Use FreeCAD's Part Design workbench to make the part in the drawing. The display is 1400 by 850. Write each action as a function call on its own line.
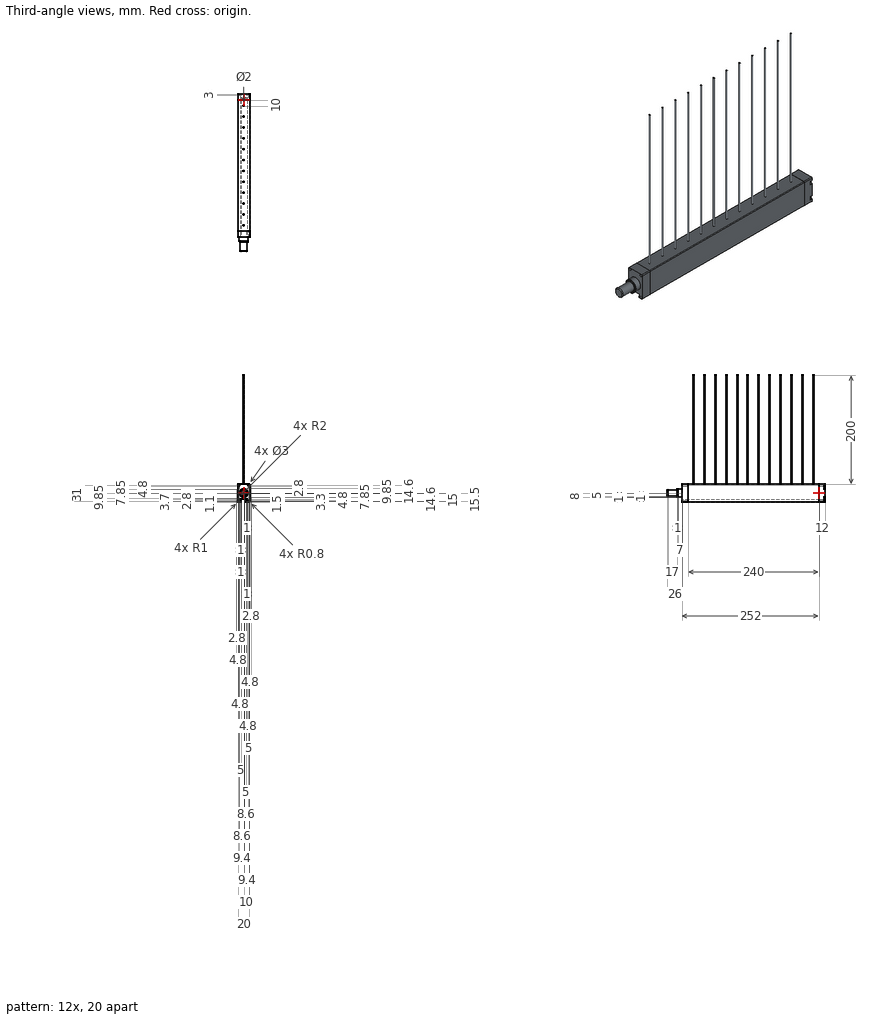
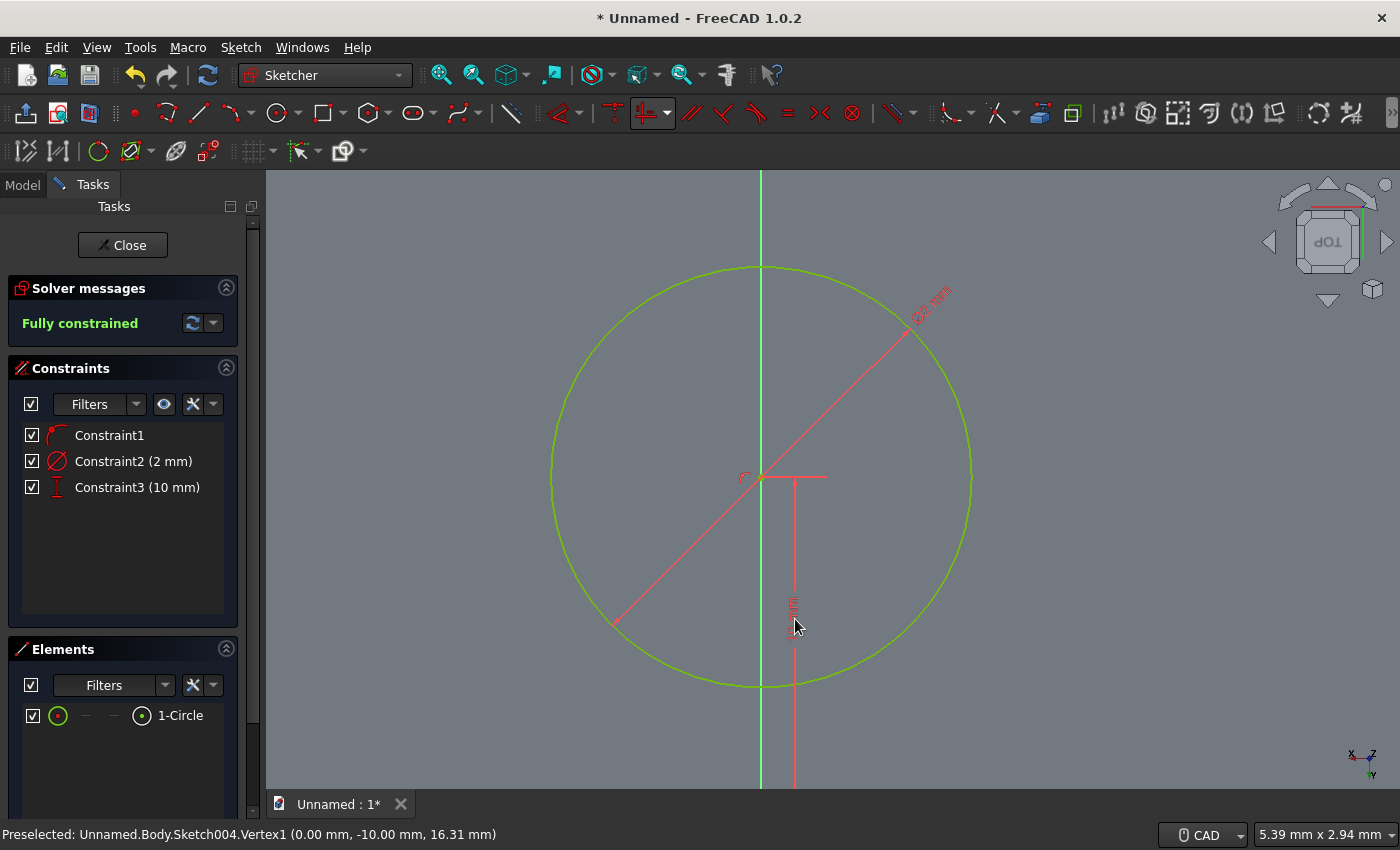
click(123, 245)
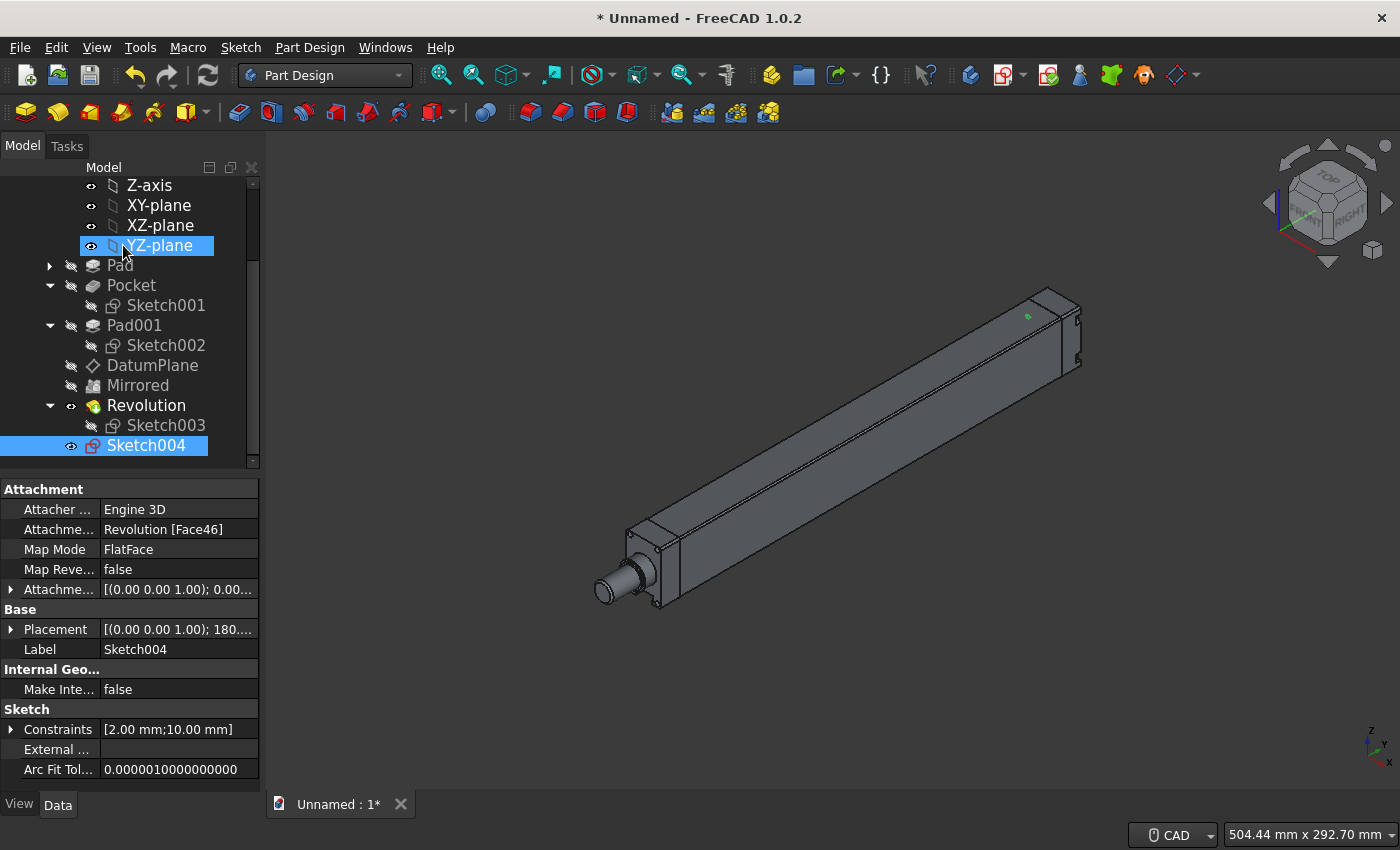
click(26, 112)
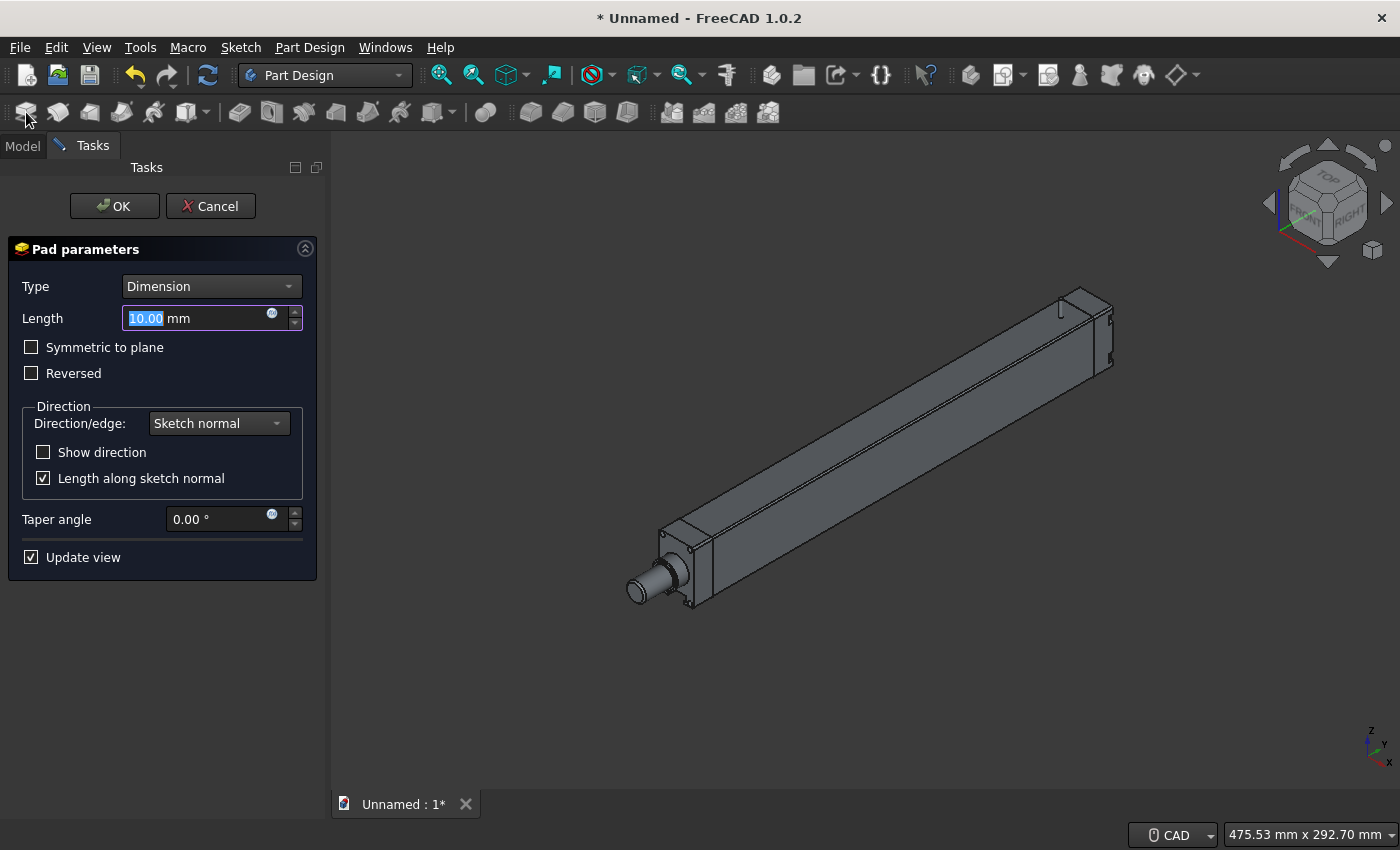
text(200)
key(Tab)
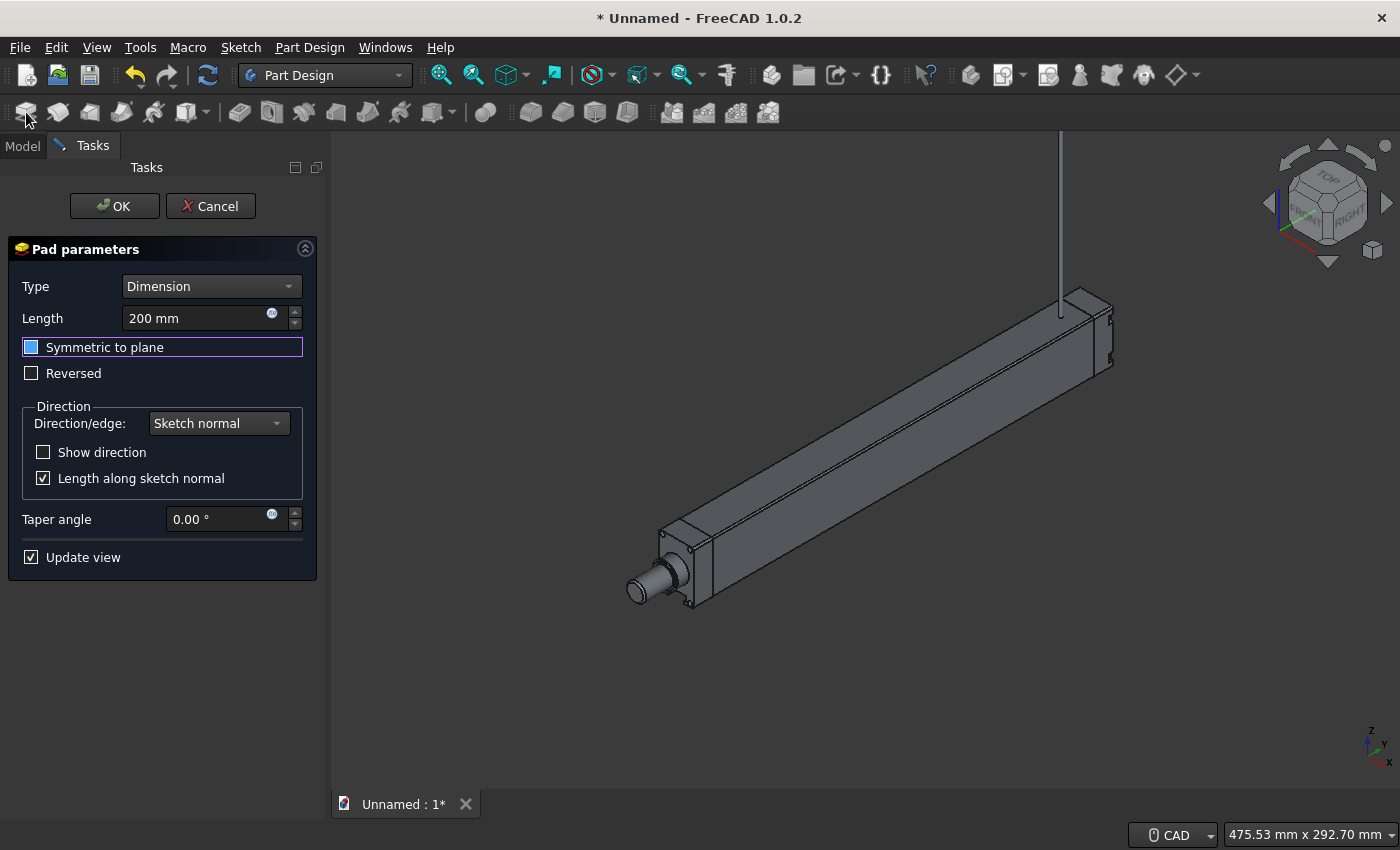
click(115, 206)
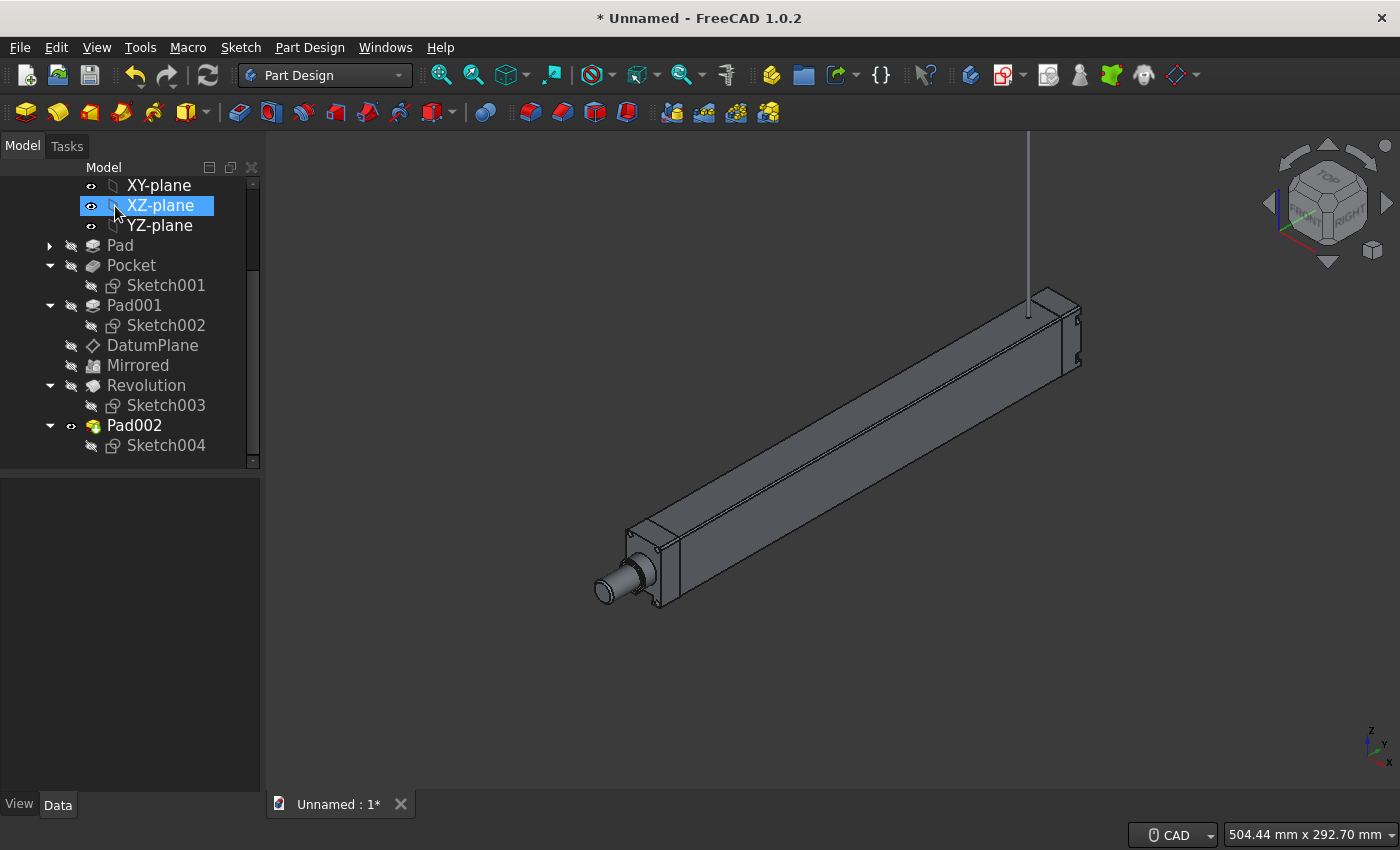
click(442, 76)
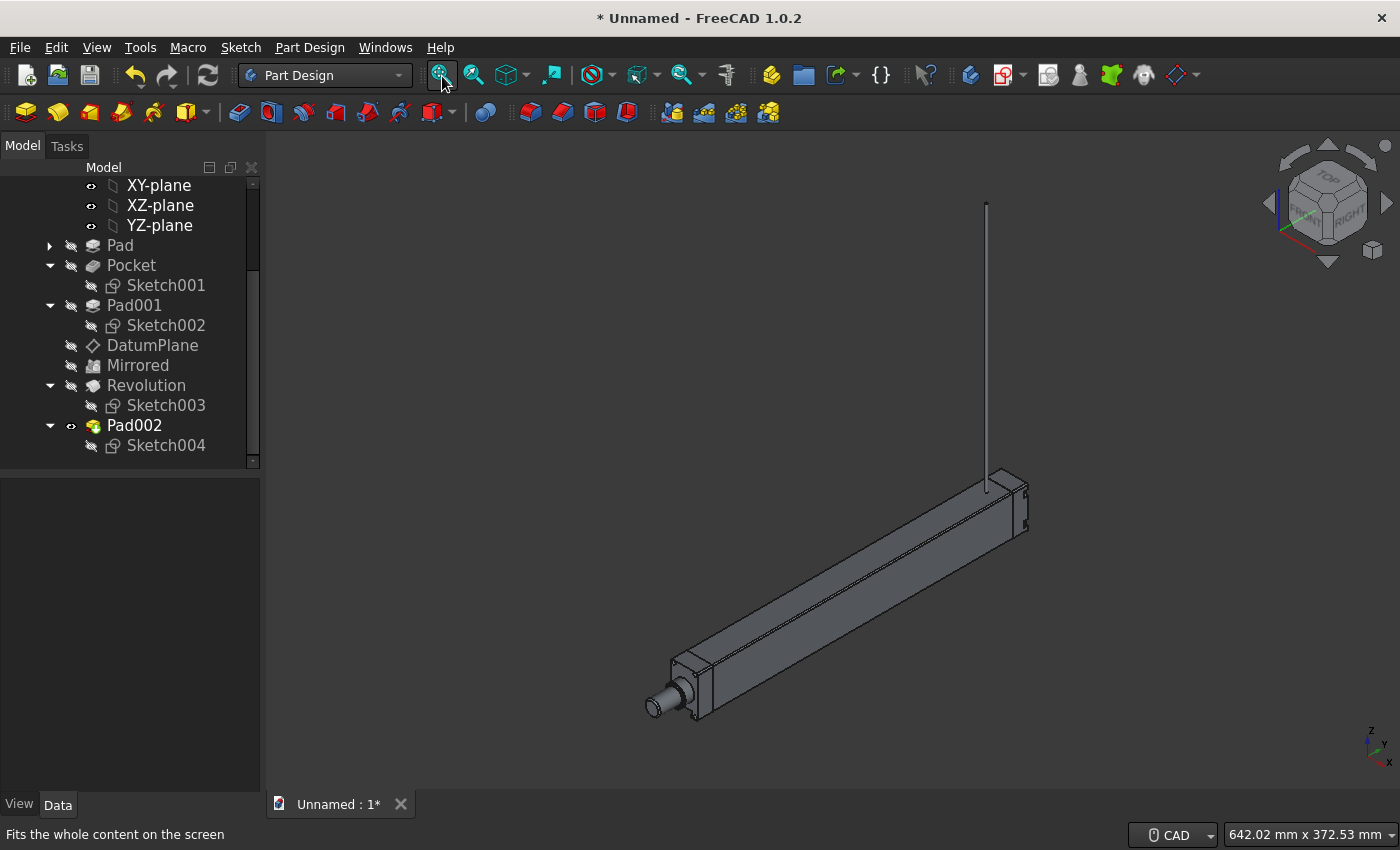
click(116, 426)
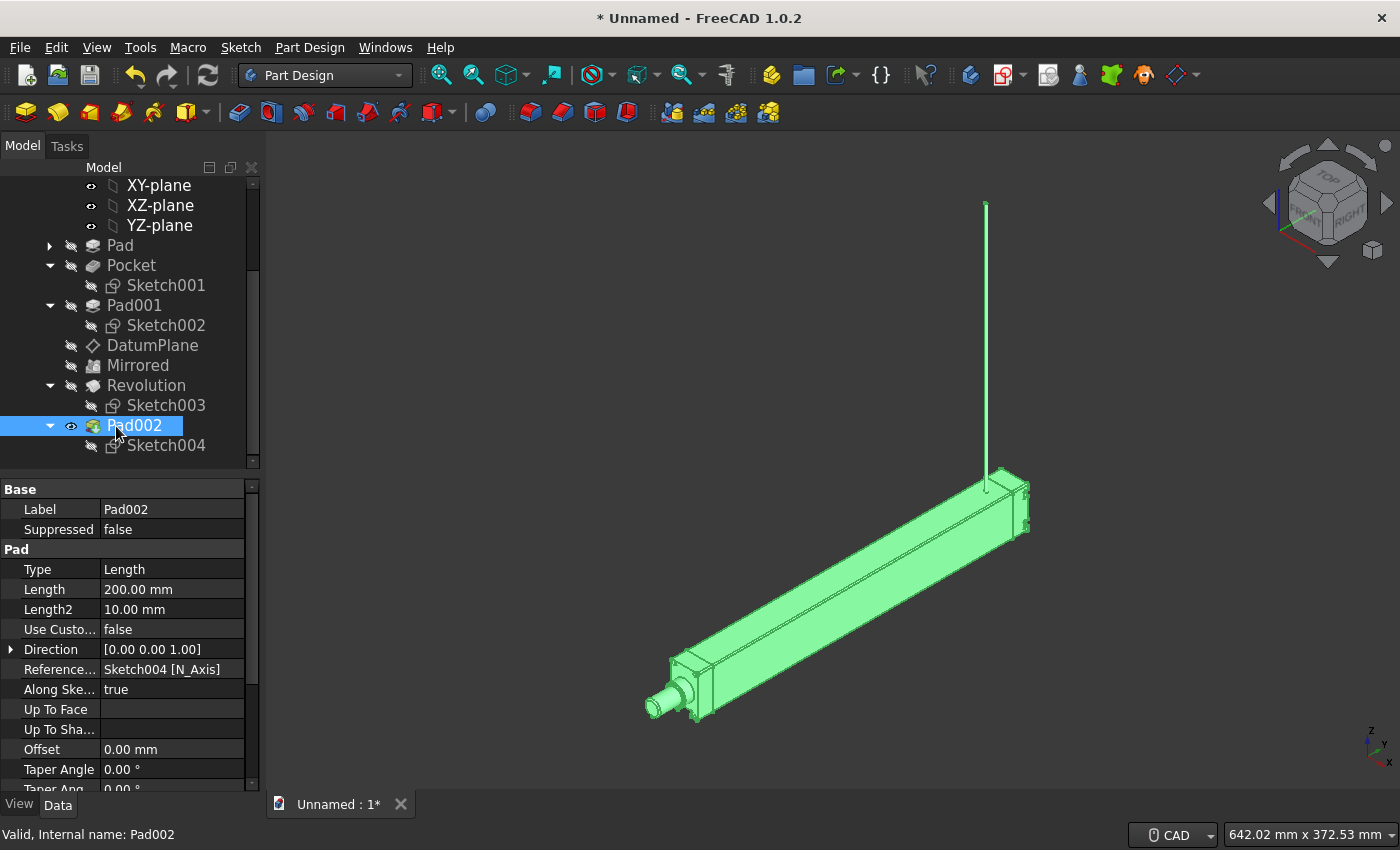
click(704, 112)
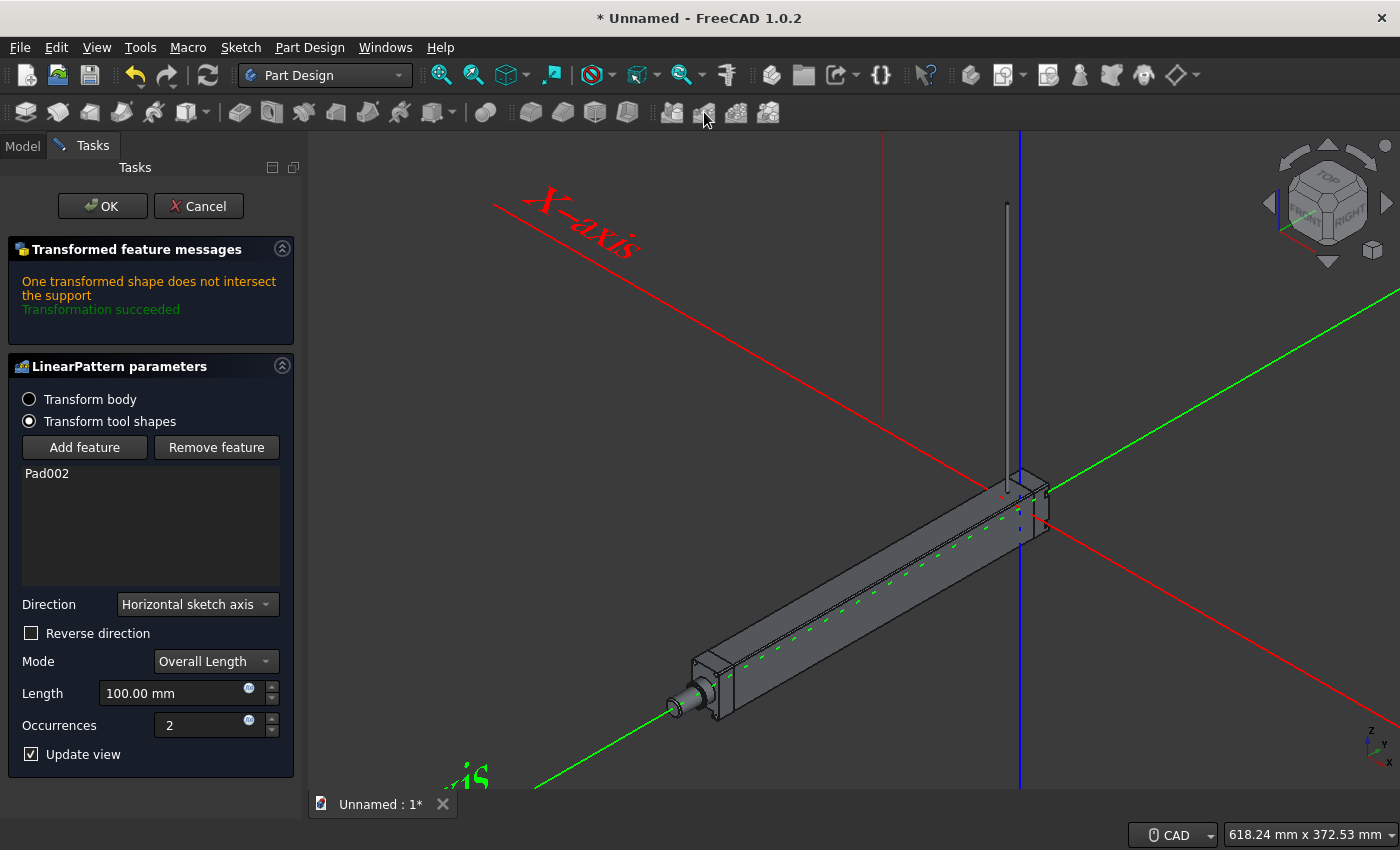
click(198, 604)